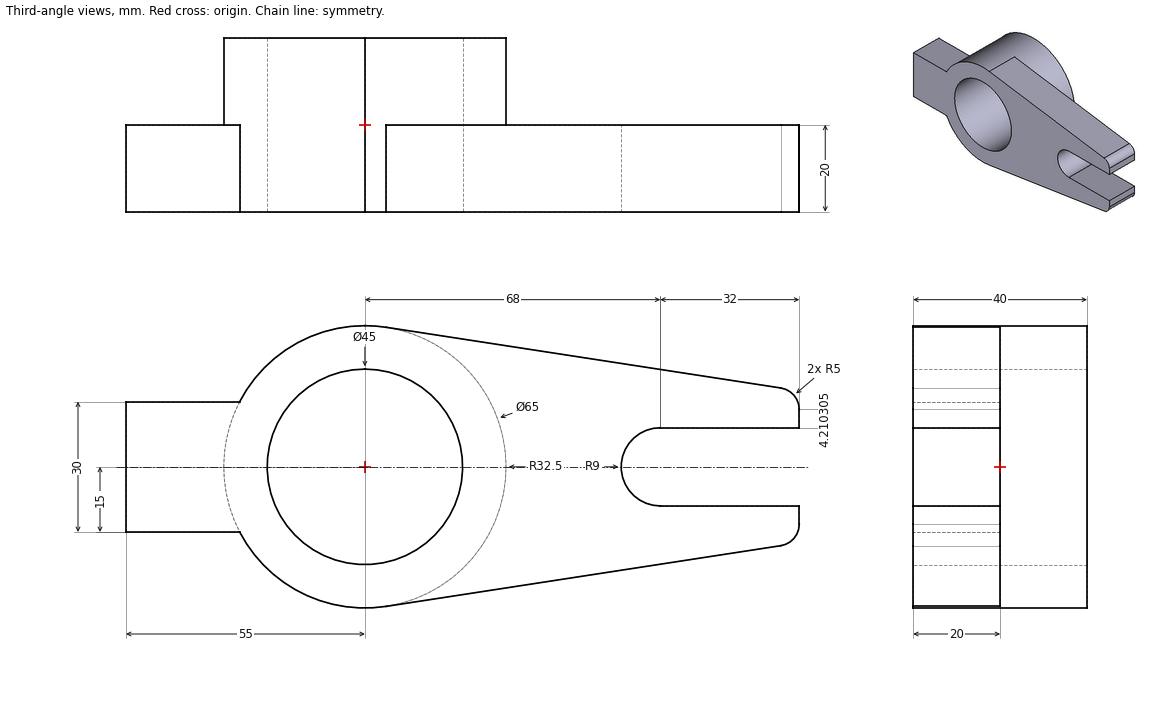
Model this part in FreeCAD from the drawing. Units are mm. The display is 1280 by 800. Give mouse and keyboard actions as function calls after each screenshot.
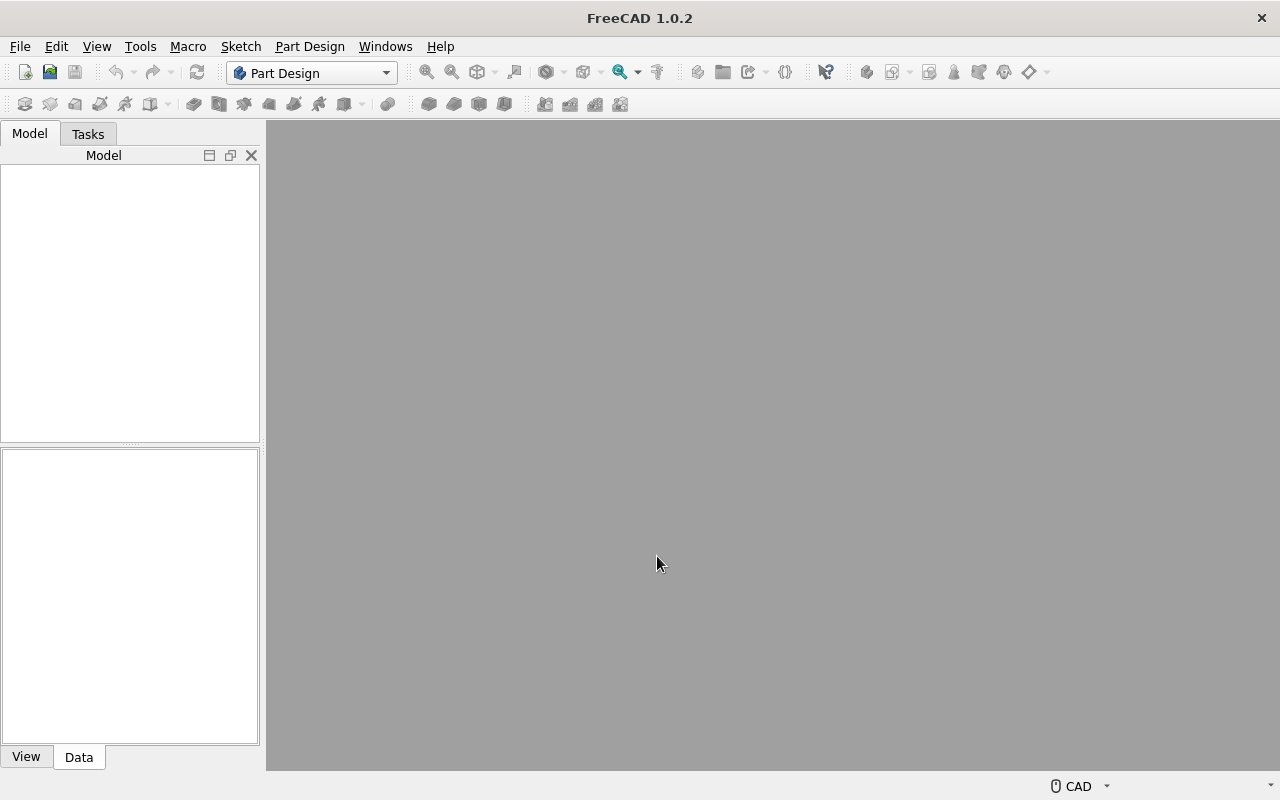
key(ctrl+n)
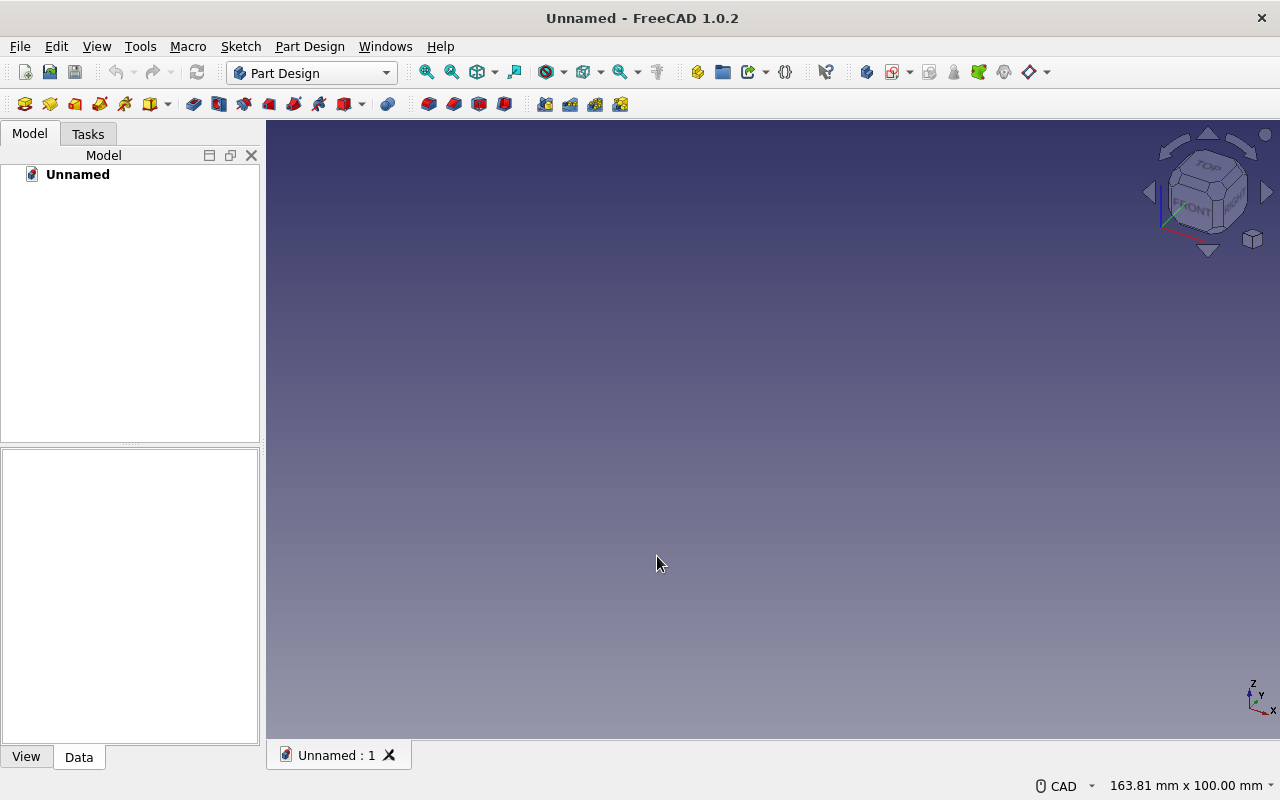
click(892, 72)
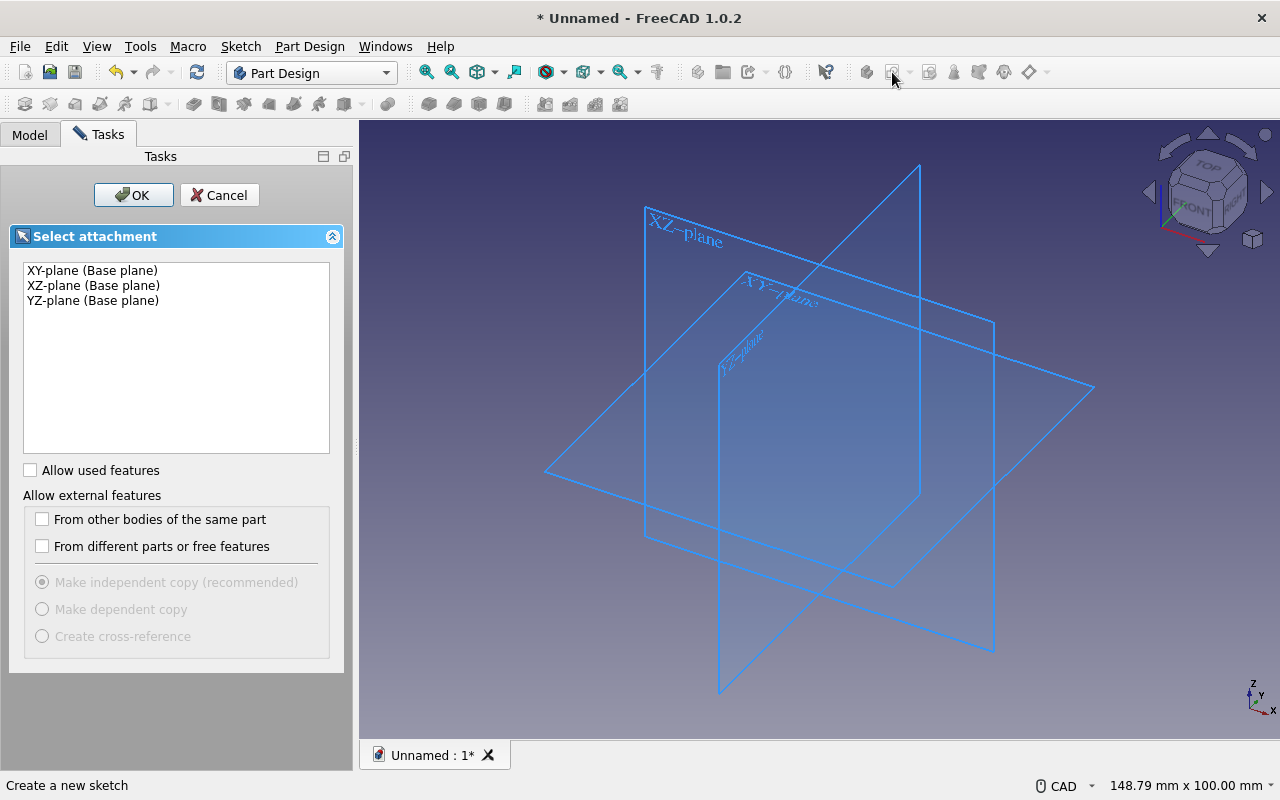
click(84, 286)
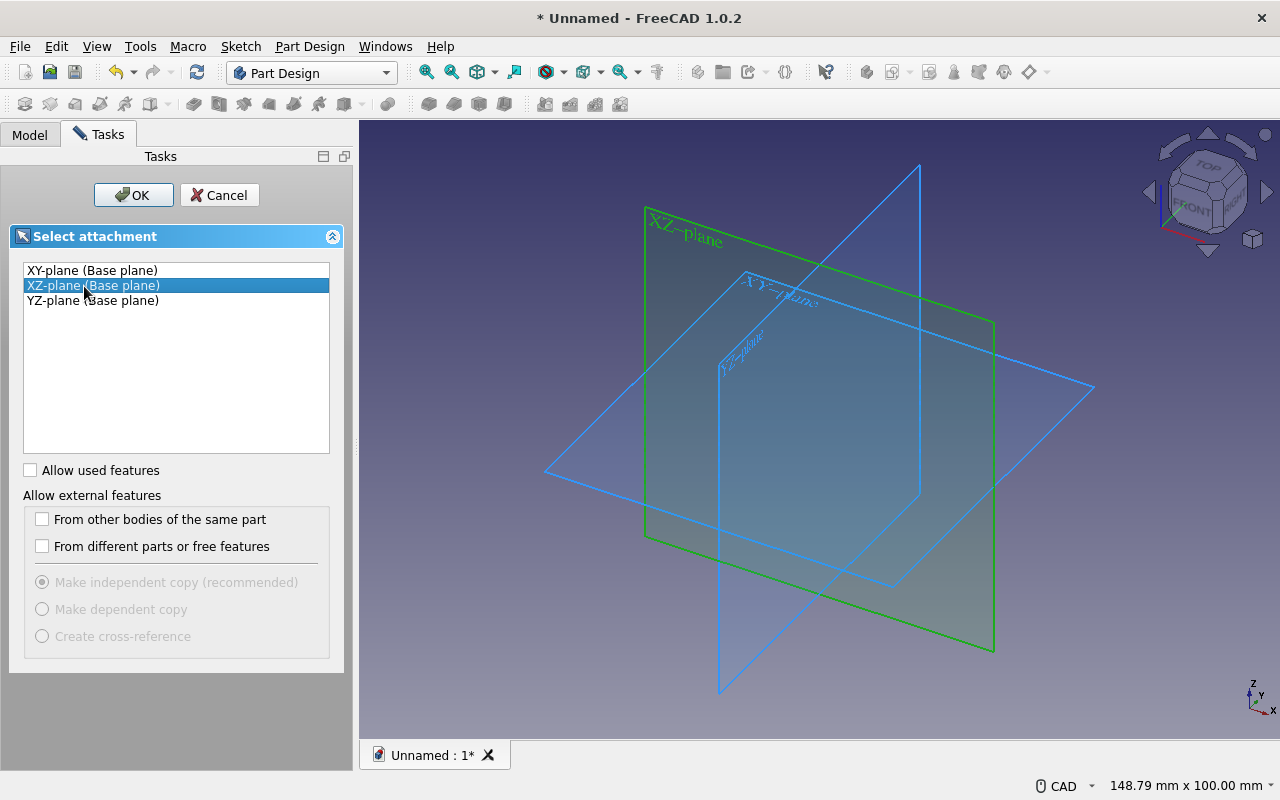
click(134, 195)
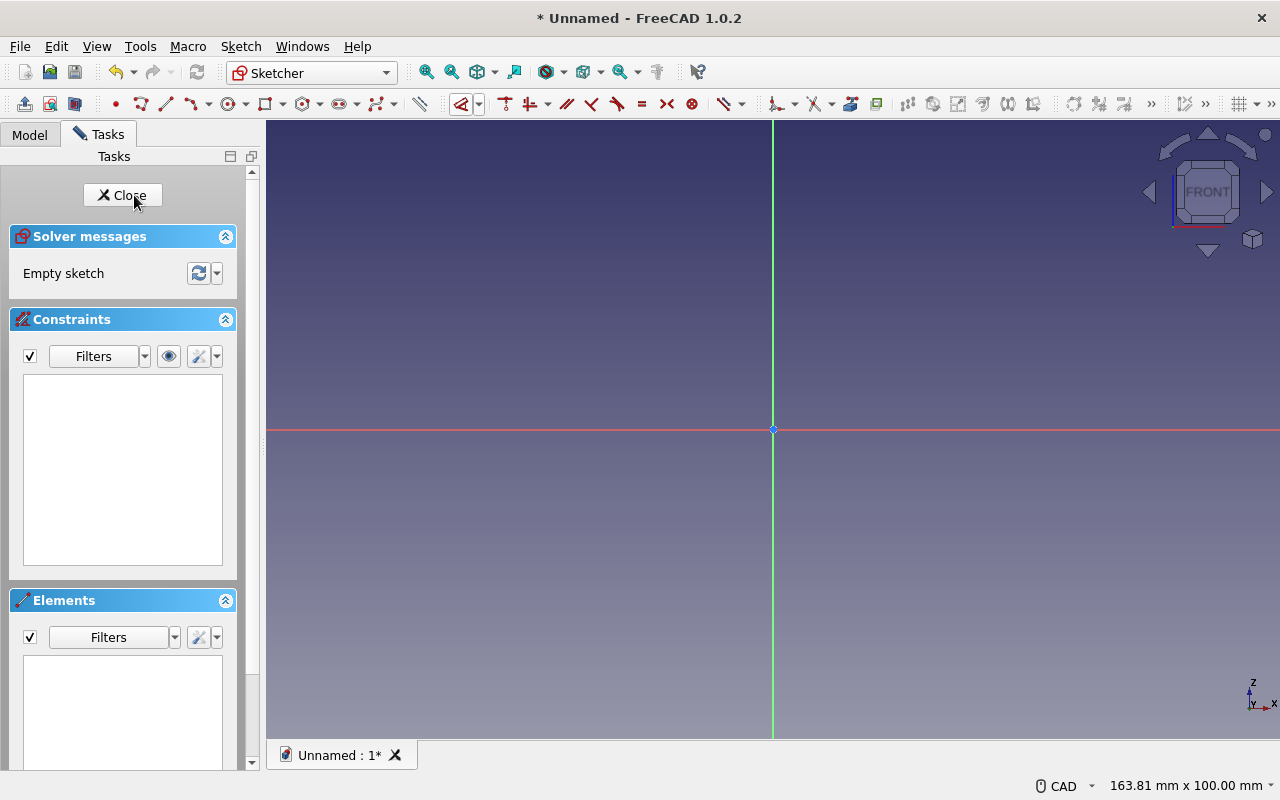
click(228, 104)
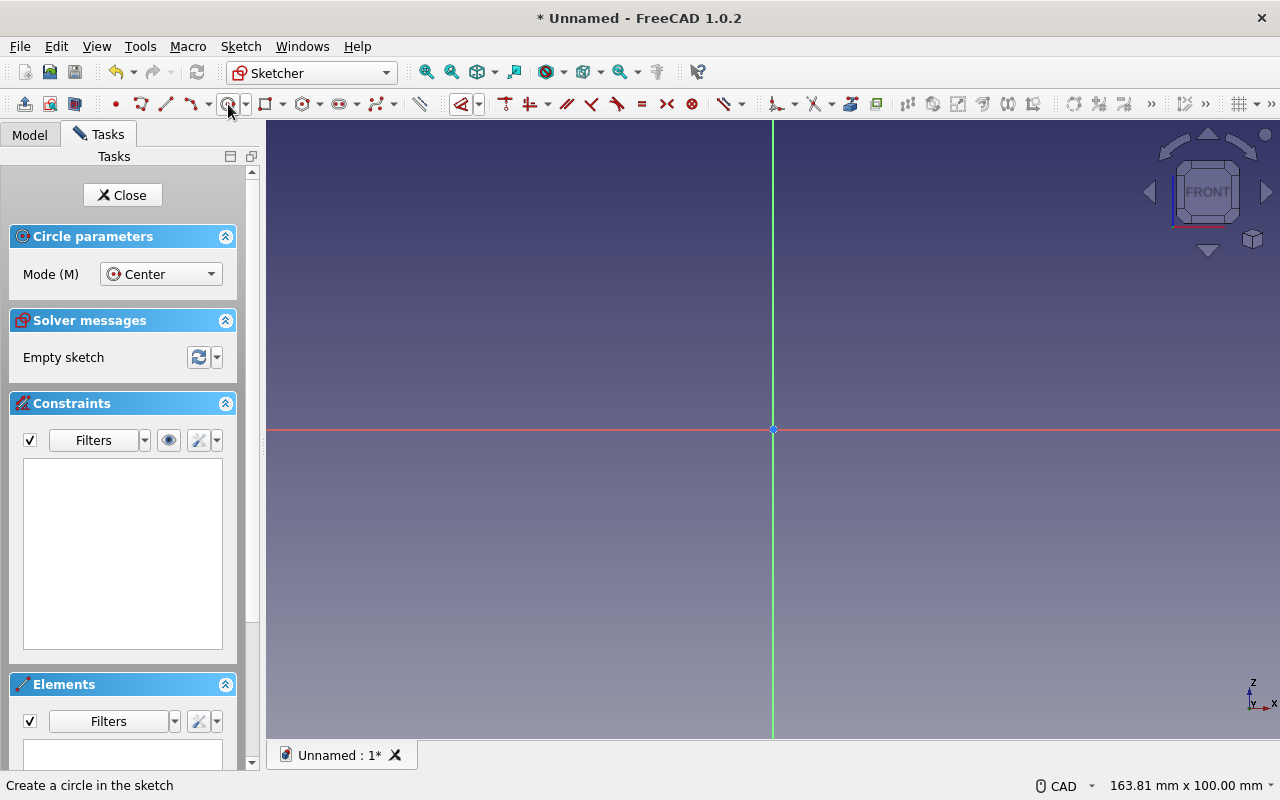
click(773, 430)
move(915, 287)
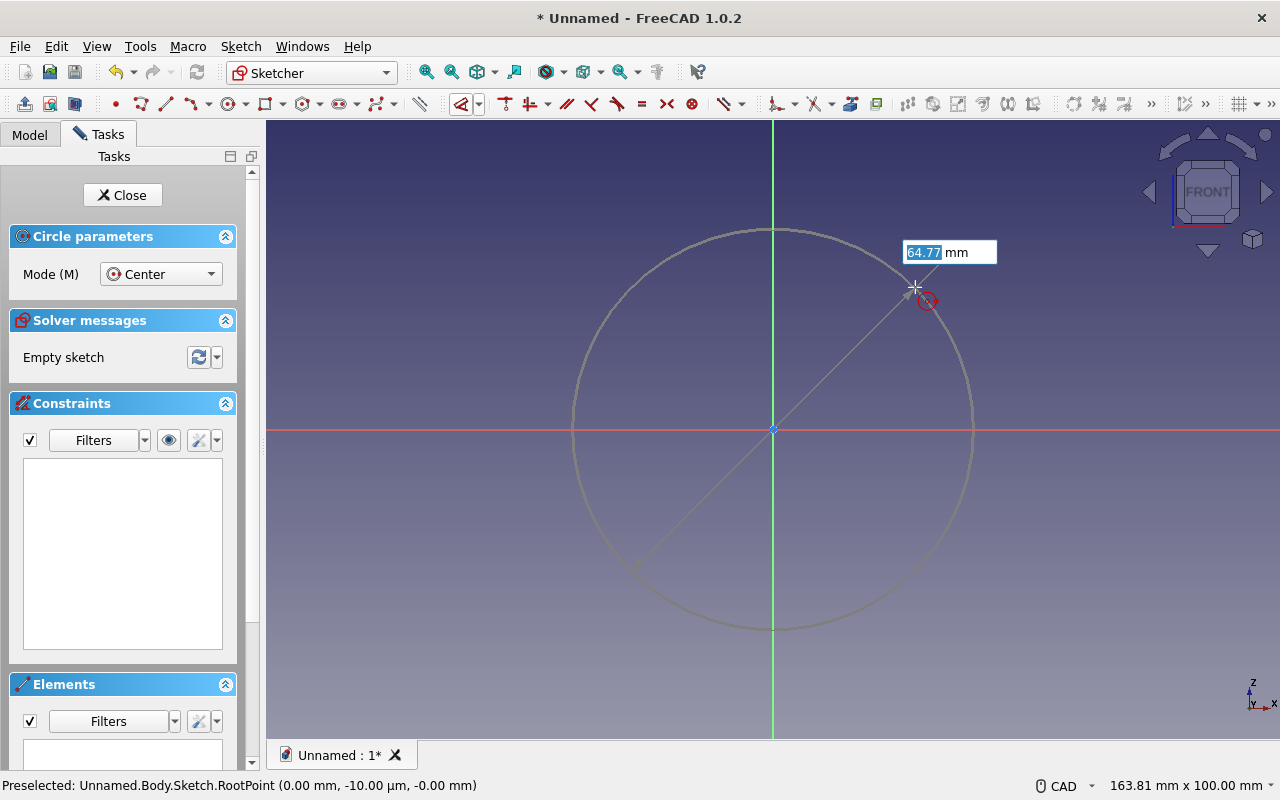
text(65)
key(Return)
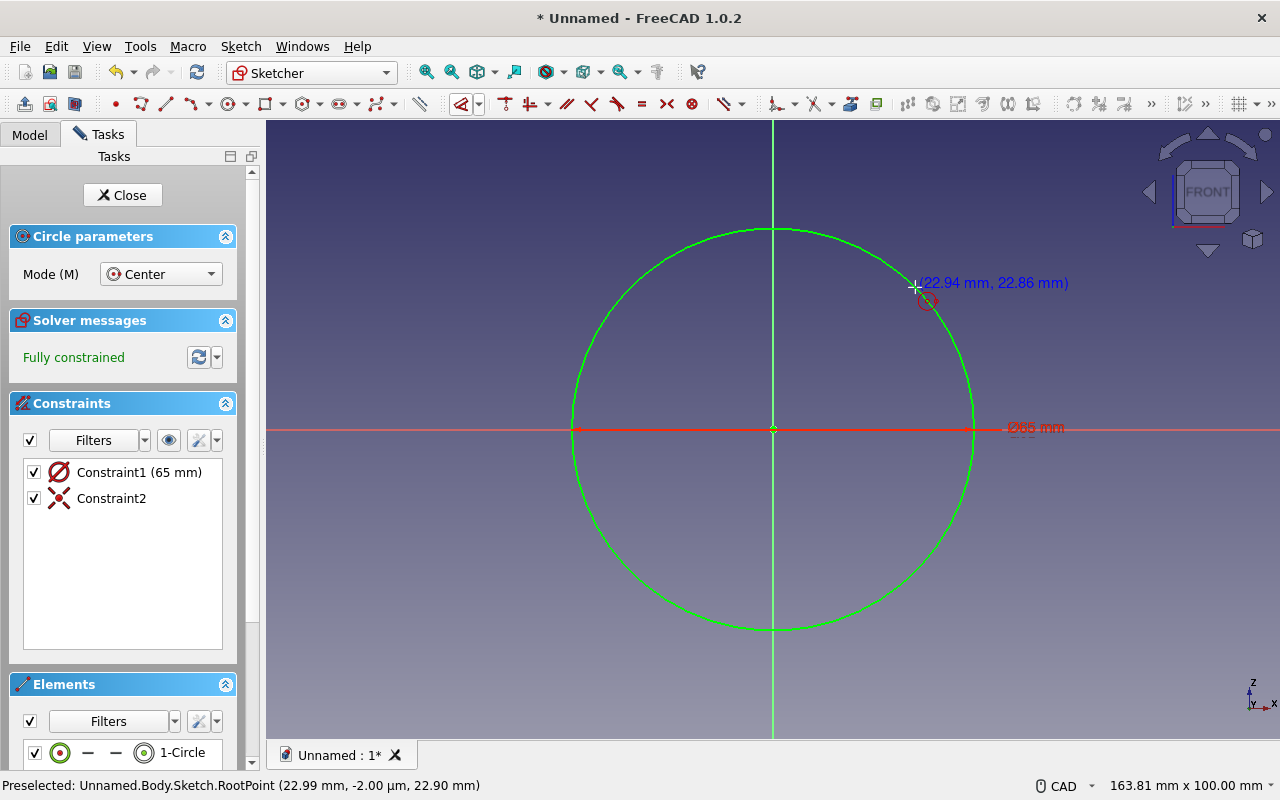
click(773, 430)
move(871, 331)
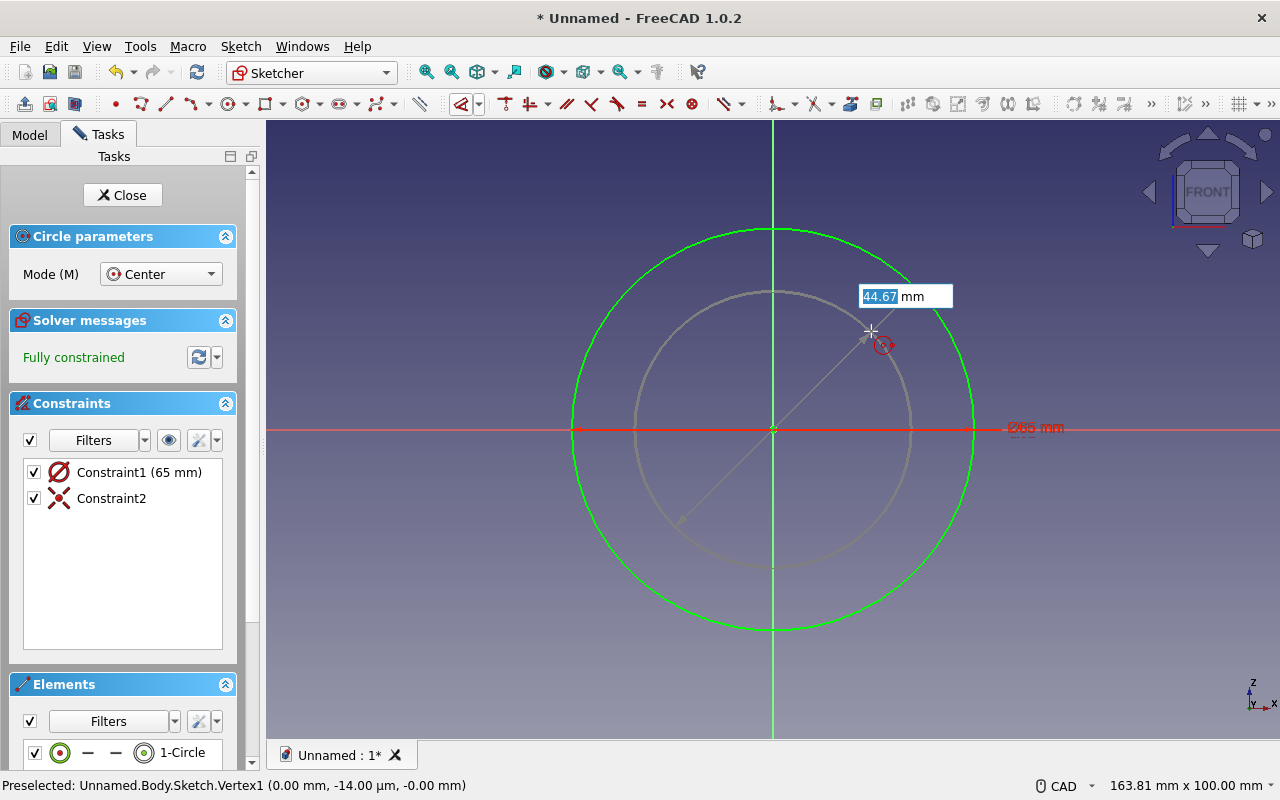
text(45)
key(Return)
key(Escape)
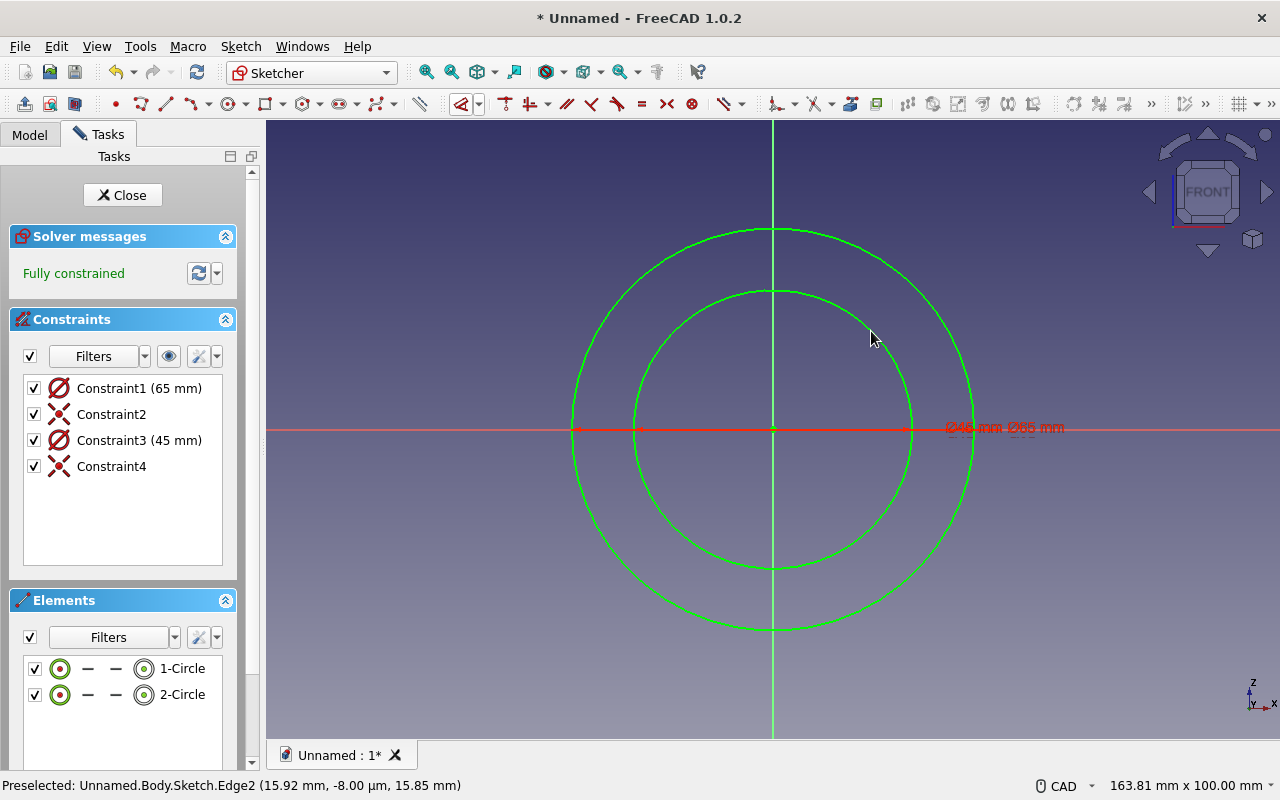
click(123, 195)